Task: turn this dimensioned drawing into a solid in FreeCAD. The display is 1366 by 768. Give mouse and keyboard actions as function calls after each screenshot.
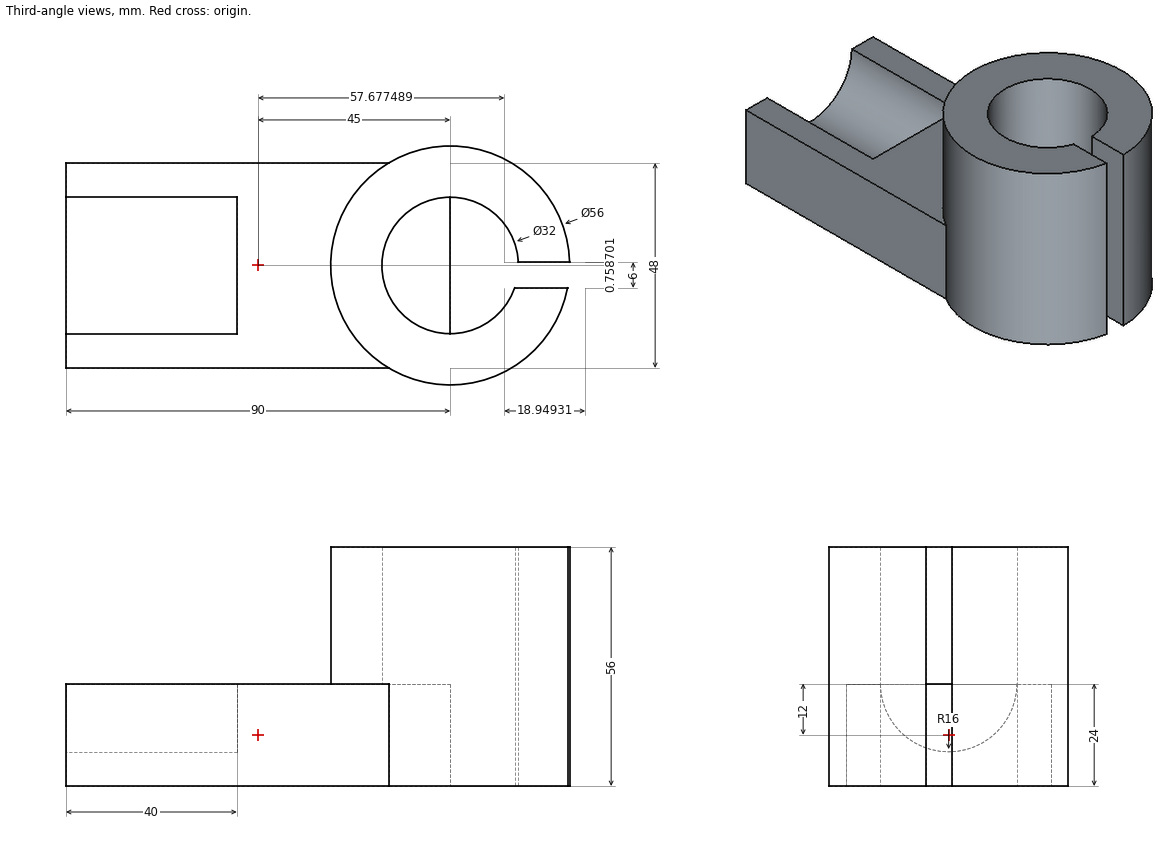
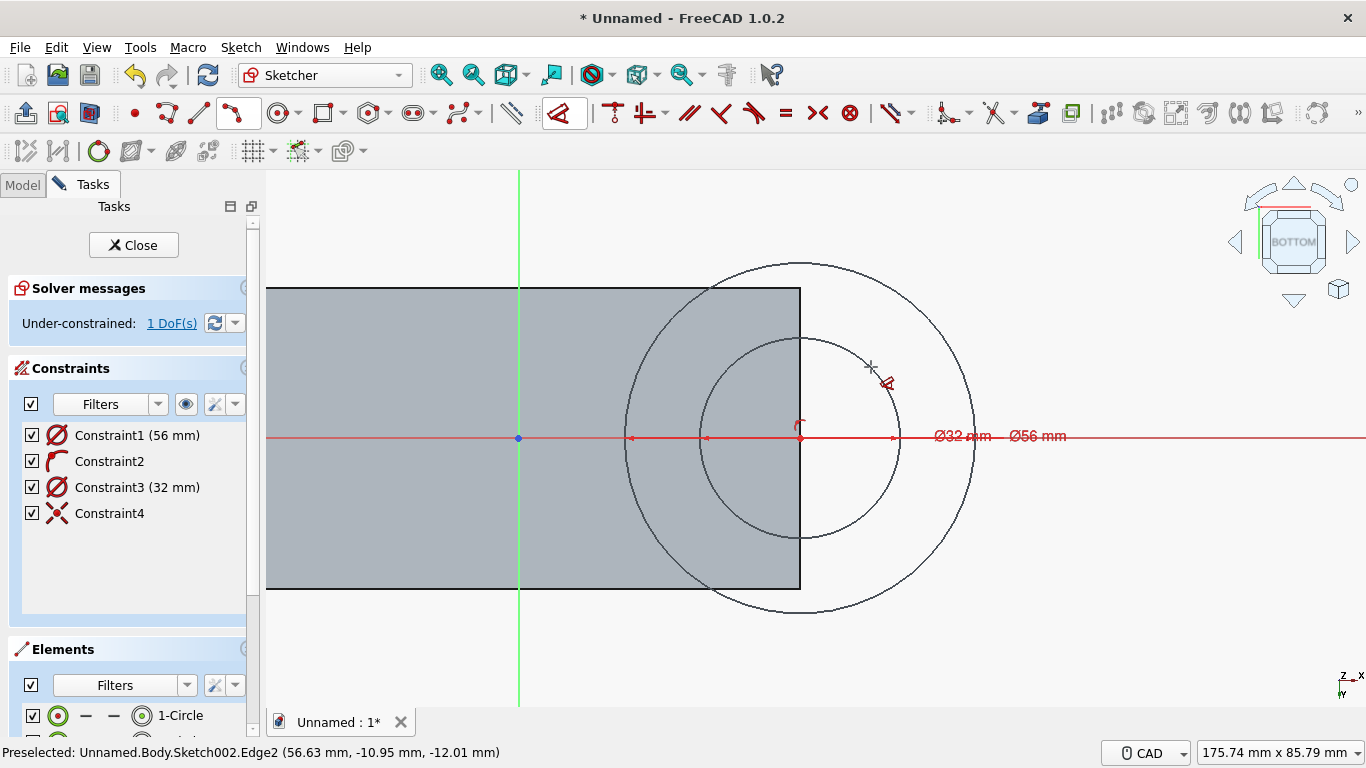
click(800, 438)
click(659, 472)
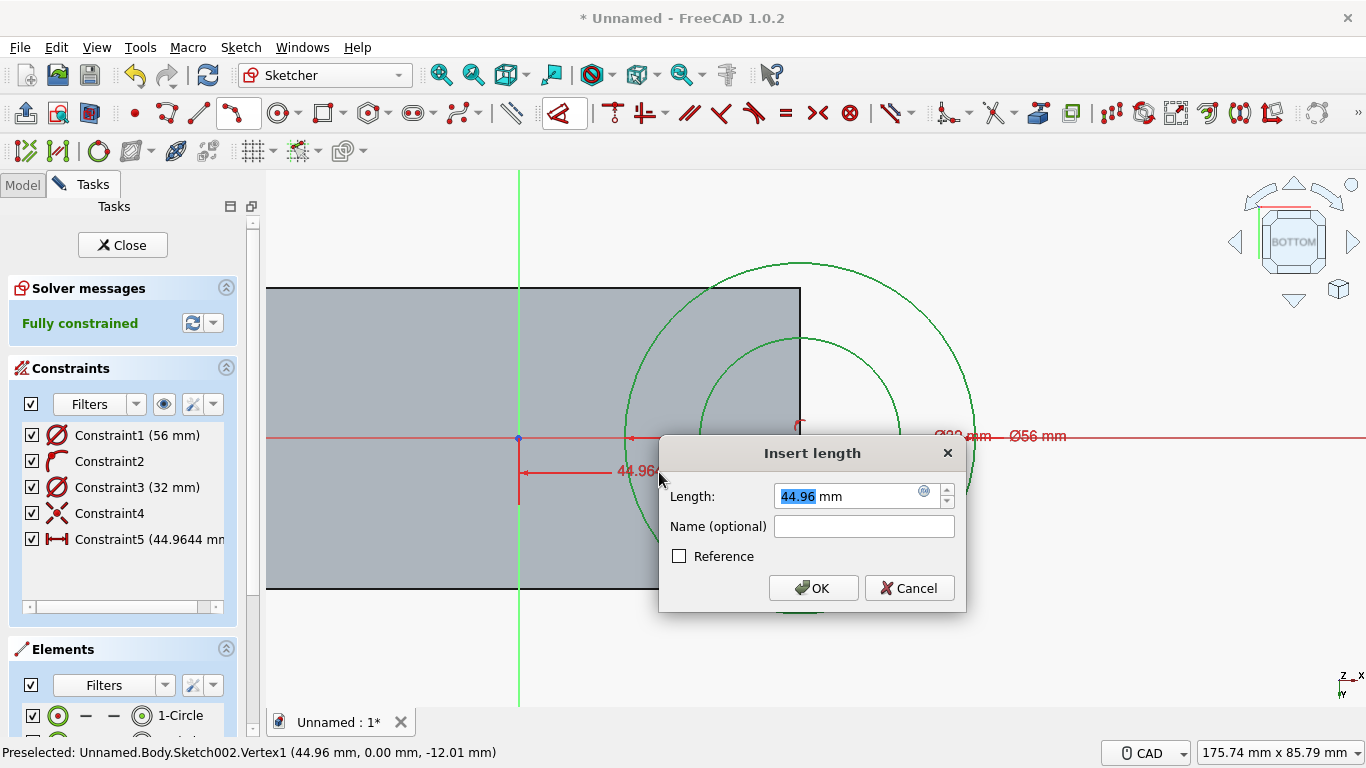
text(45)
key(Return)
key(Escape)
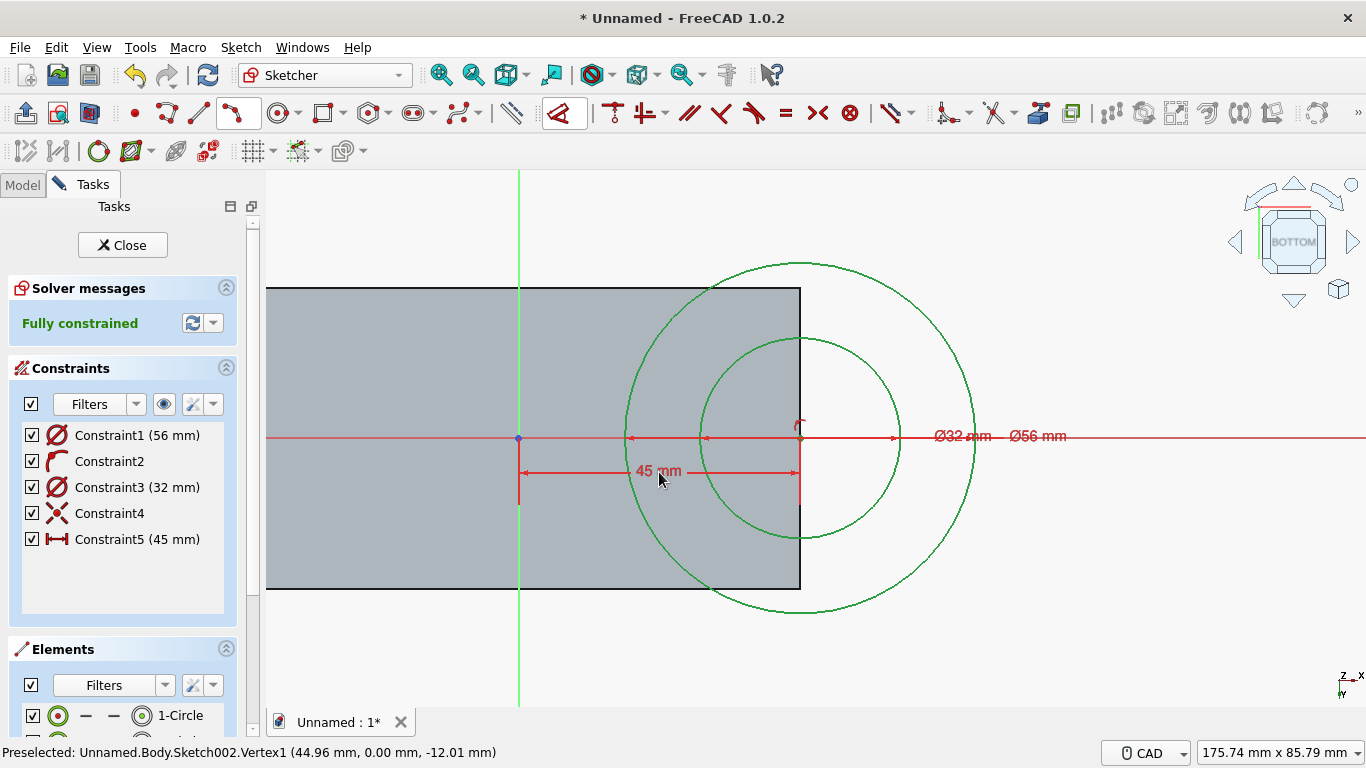
click(123, 245)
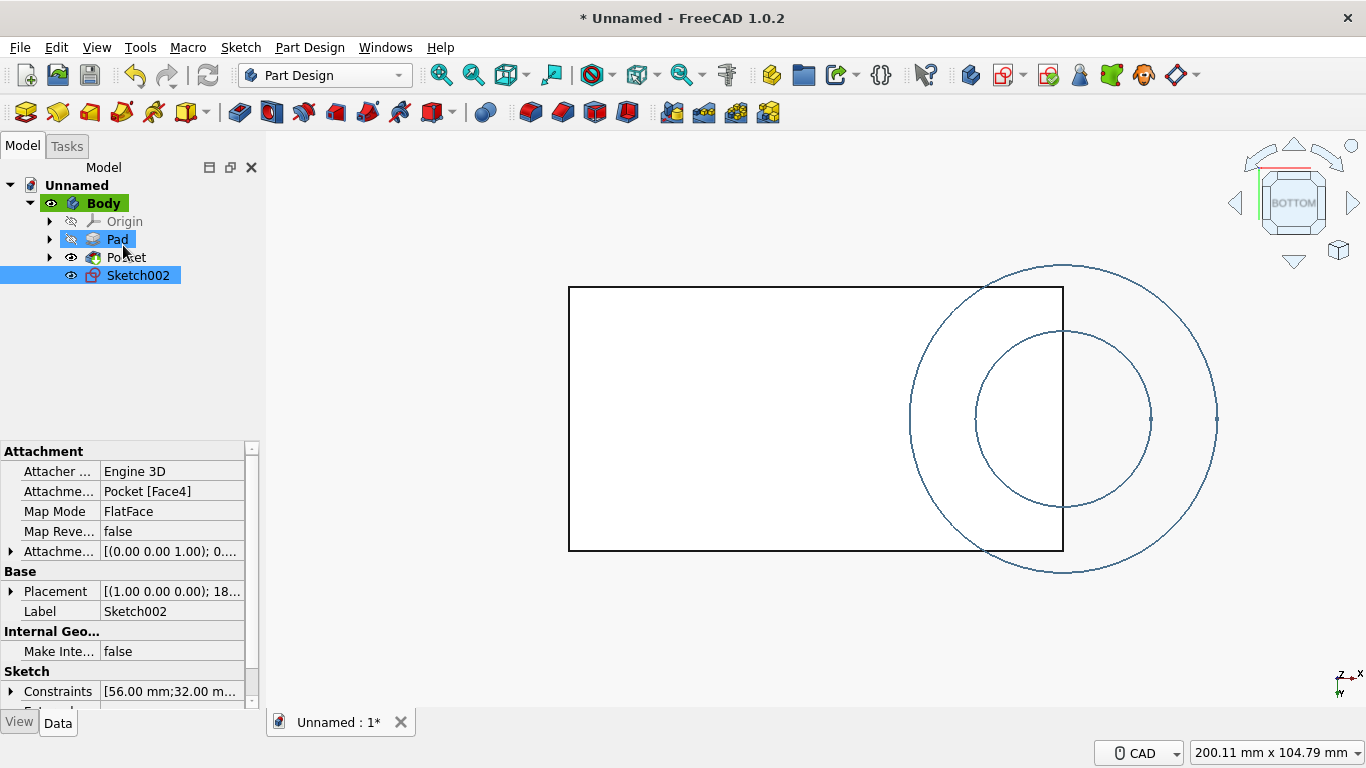
click(26, 112)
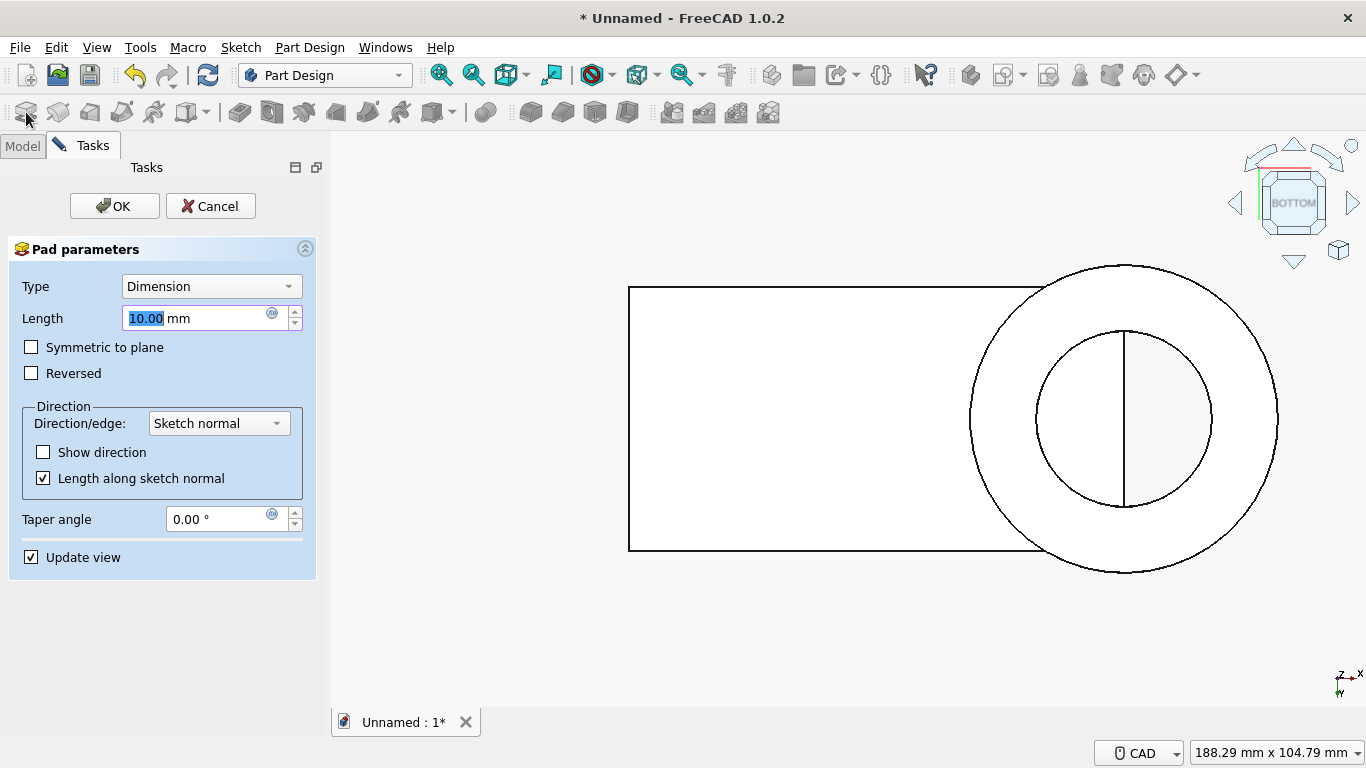
text(56)
key(Tab)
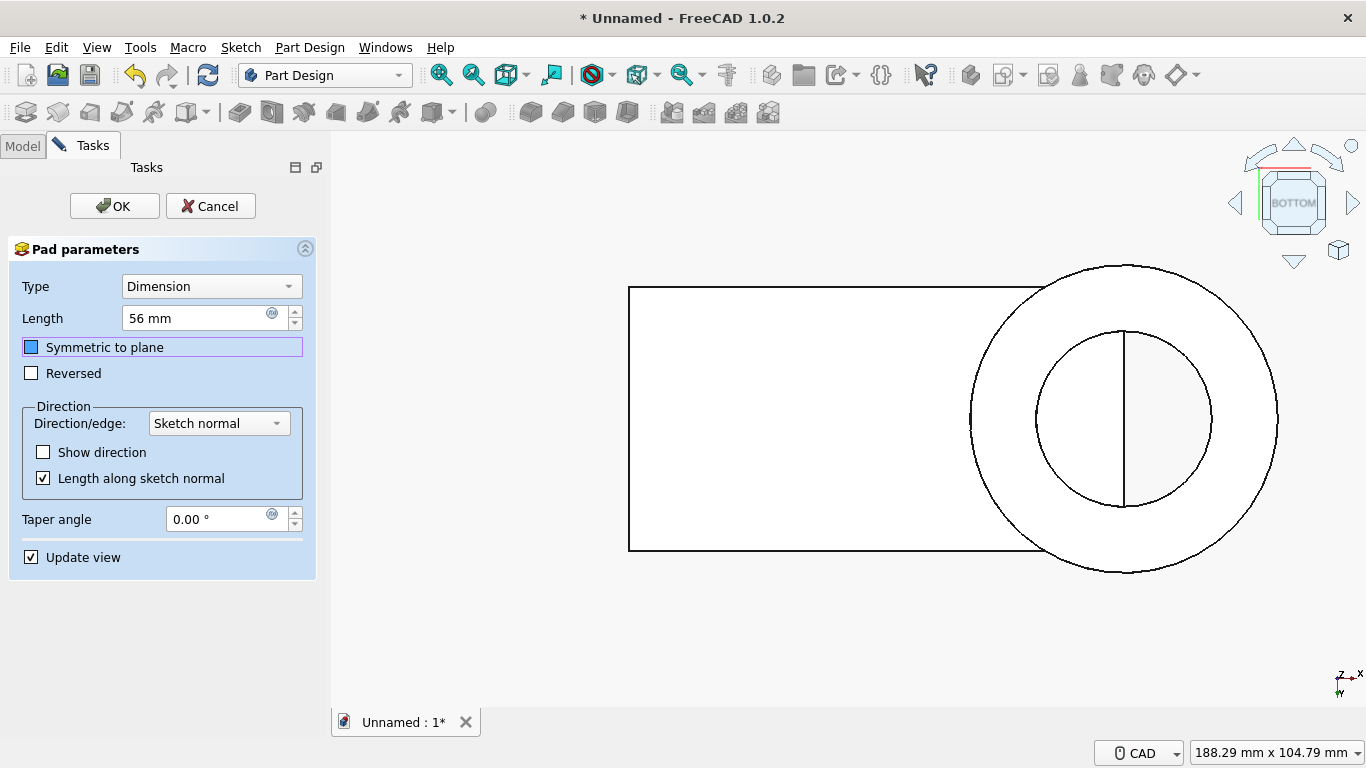
click(30, 373)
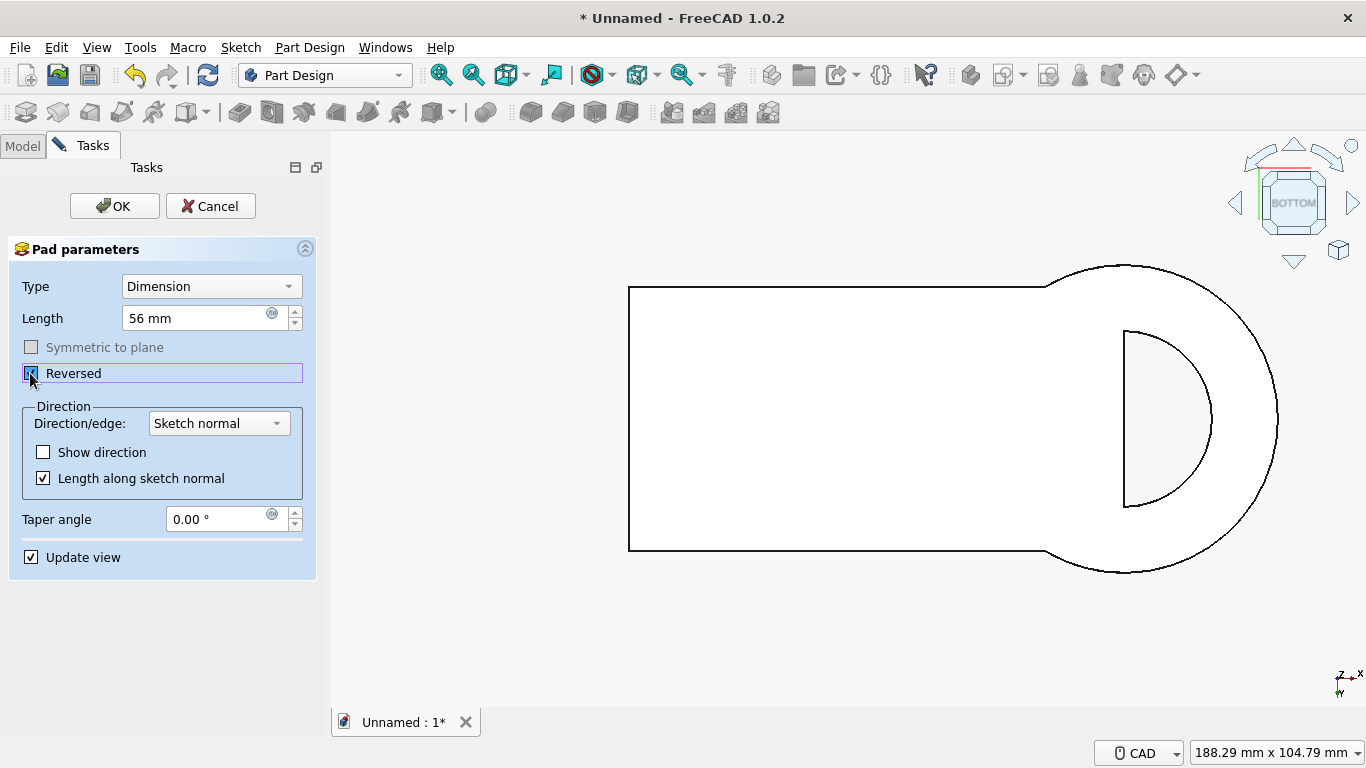
click(115, 206)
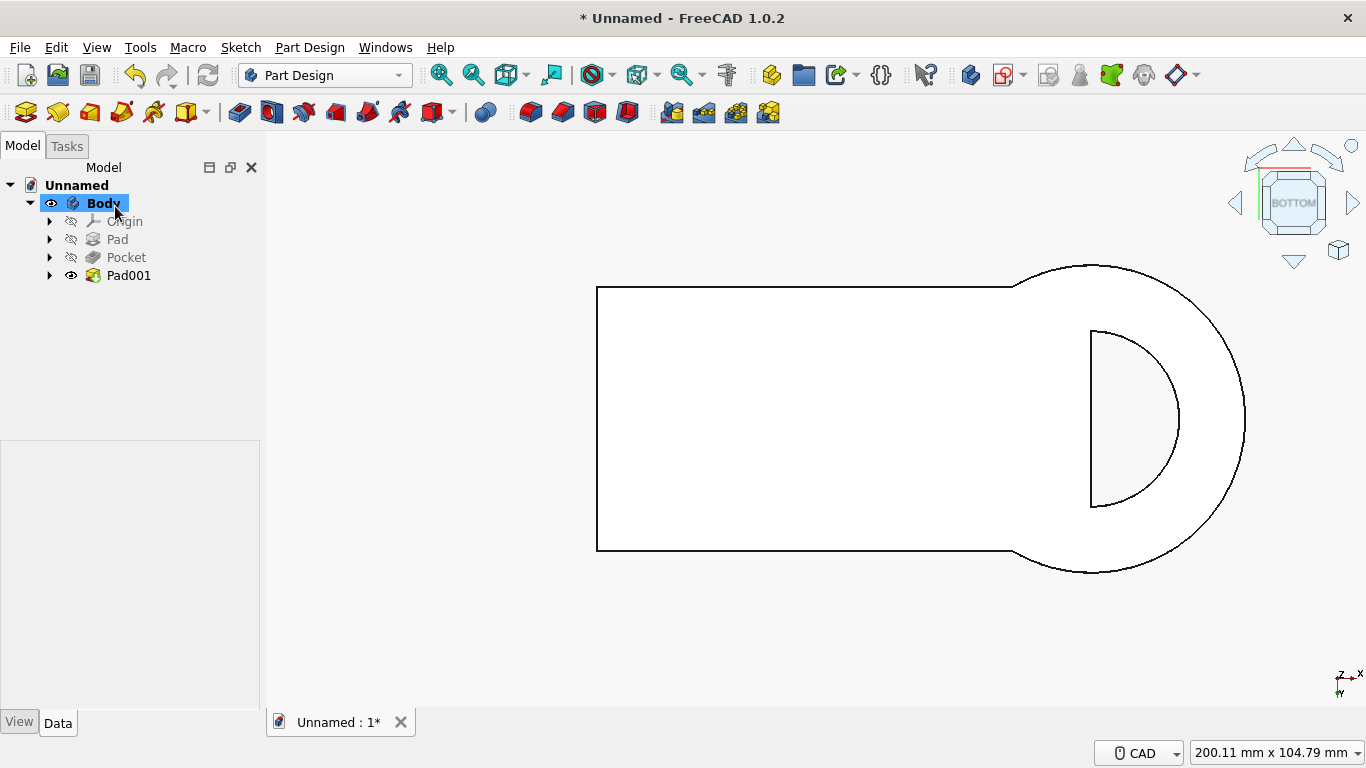
key(0)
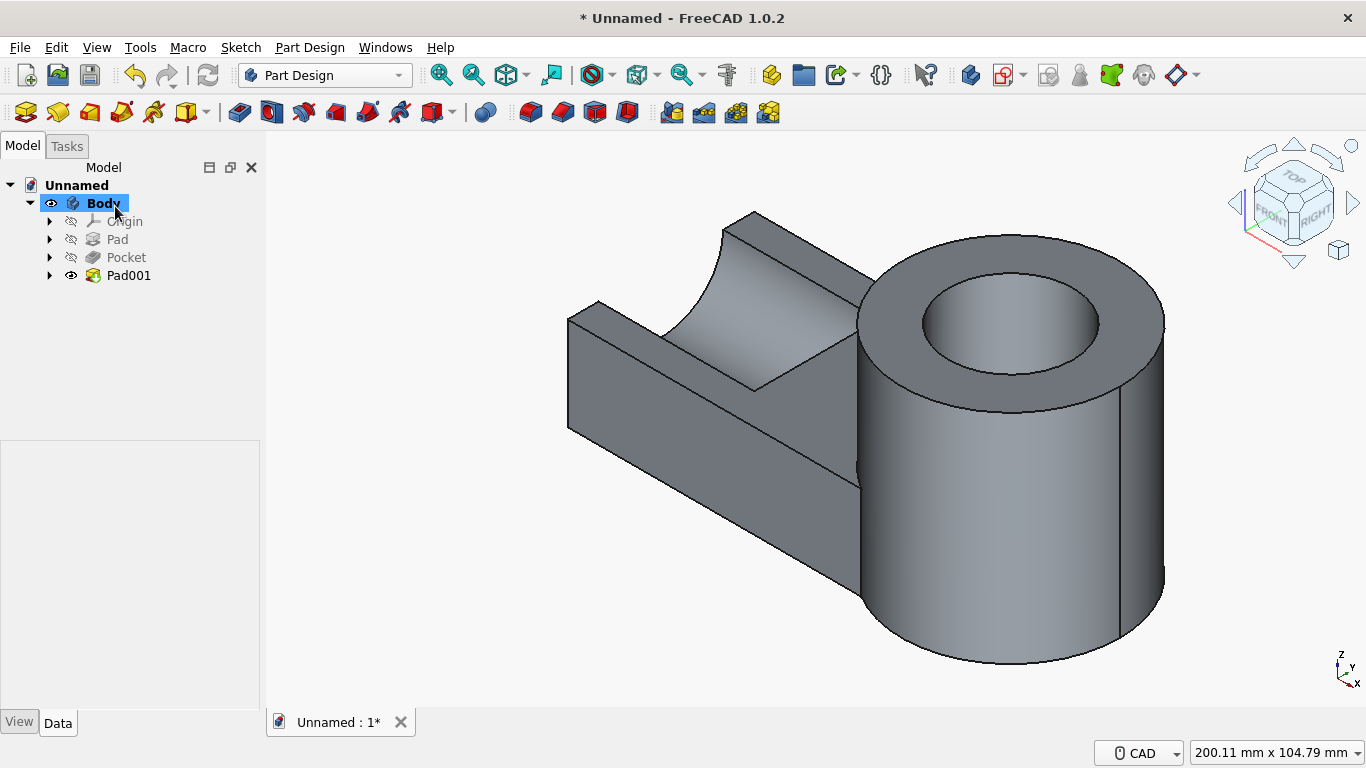
key(v)
key(f)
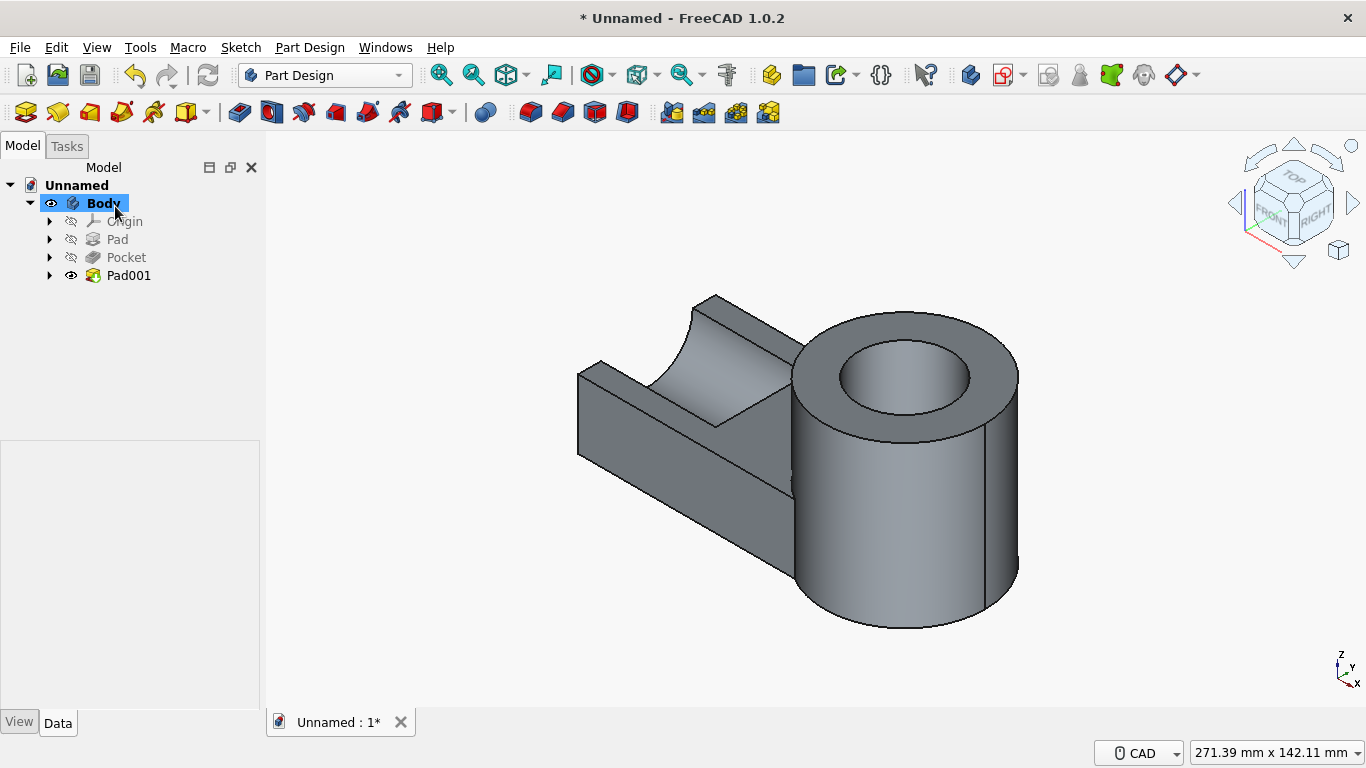
click(905, 324)